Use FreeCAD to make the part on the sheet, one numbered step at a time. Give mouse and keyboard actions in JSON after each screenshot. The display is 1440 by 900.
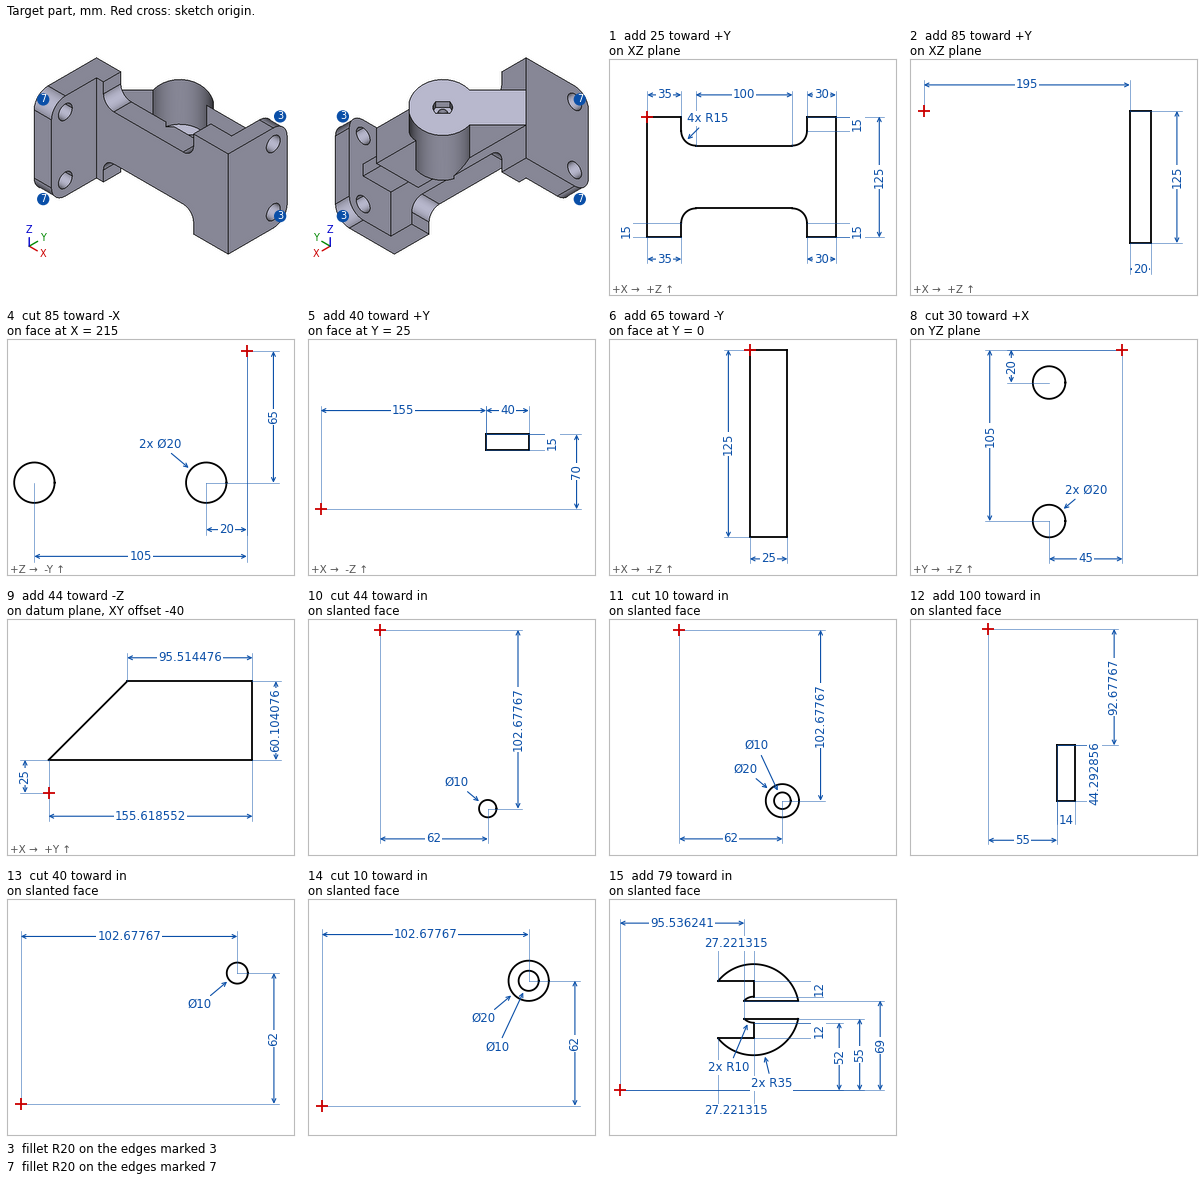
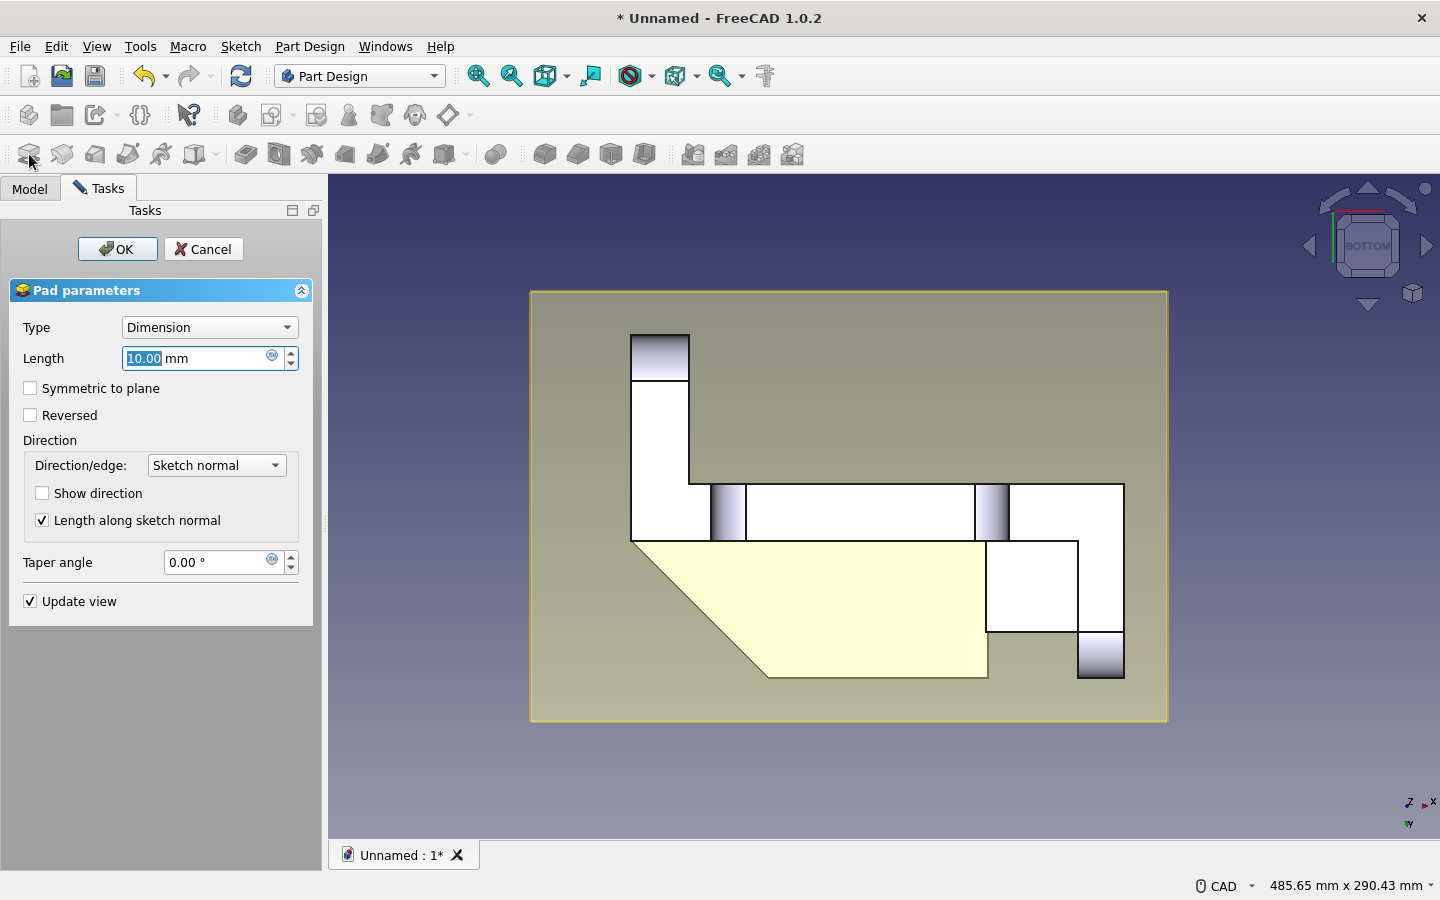
{"action": "type", "text": "44"}
{"action": "key", "text": "Tab"}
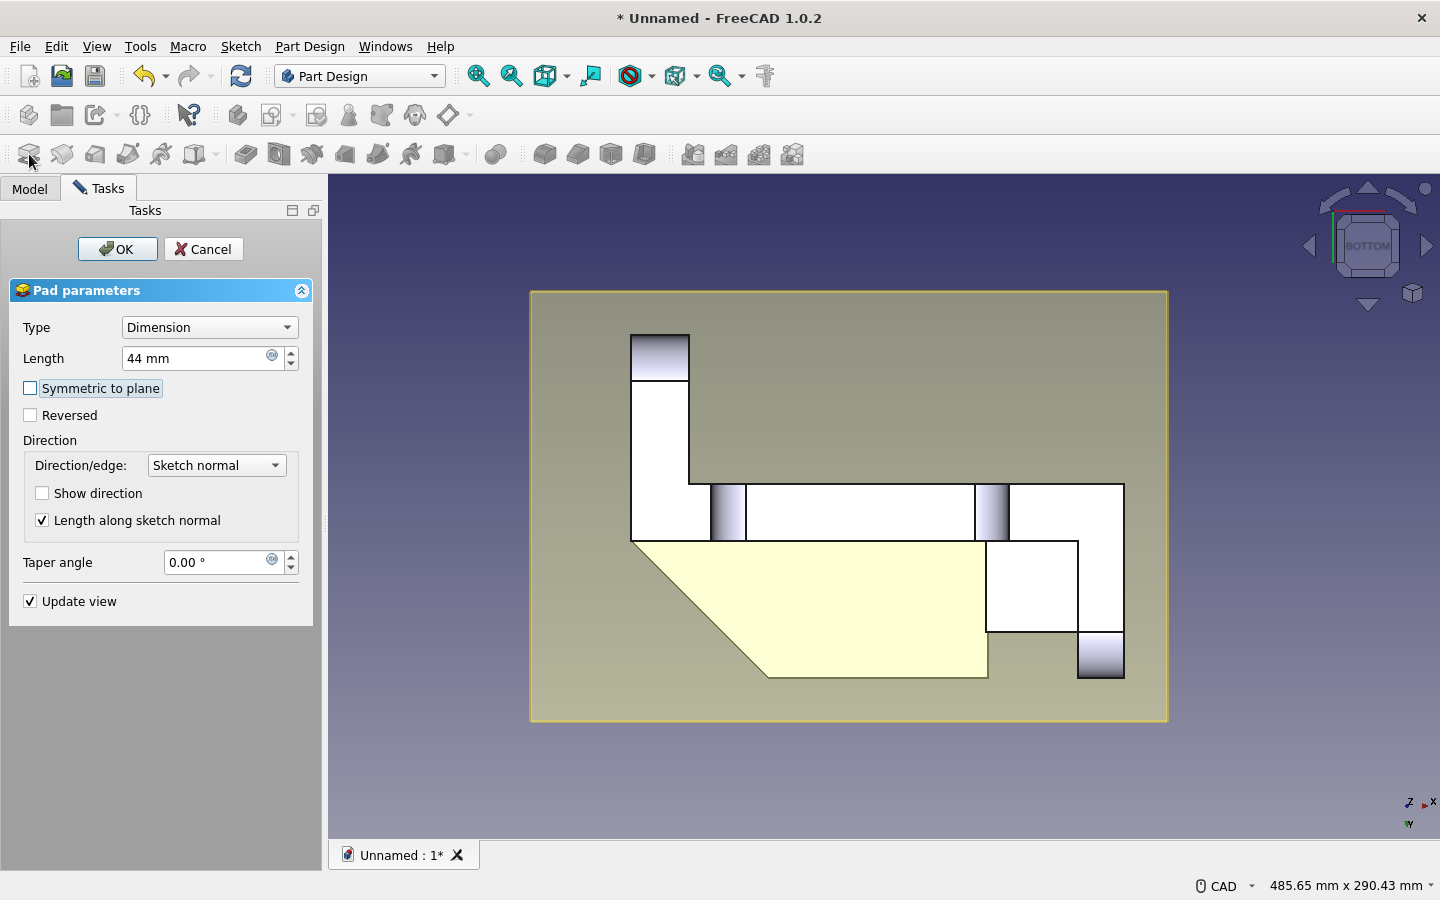
{"action": "left_click", "coordinate": [31, 415]}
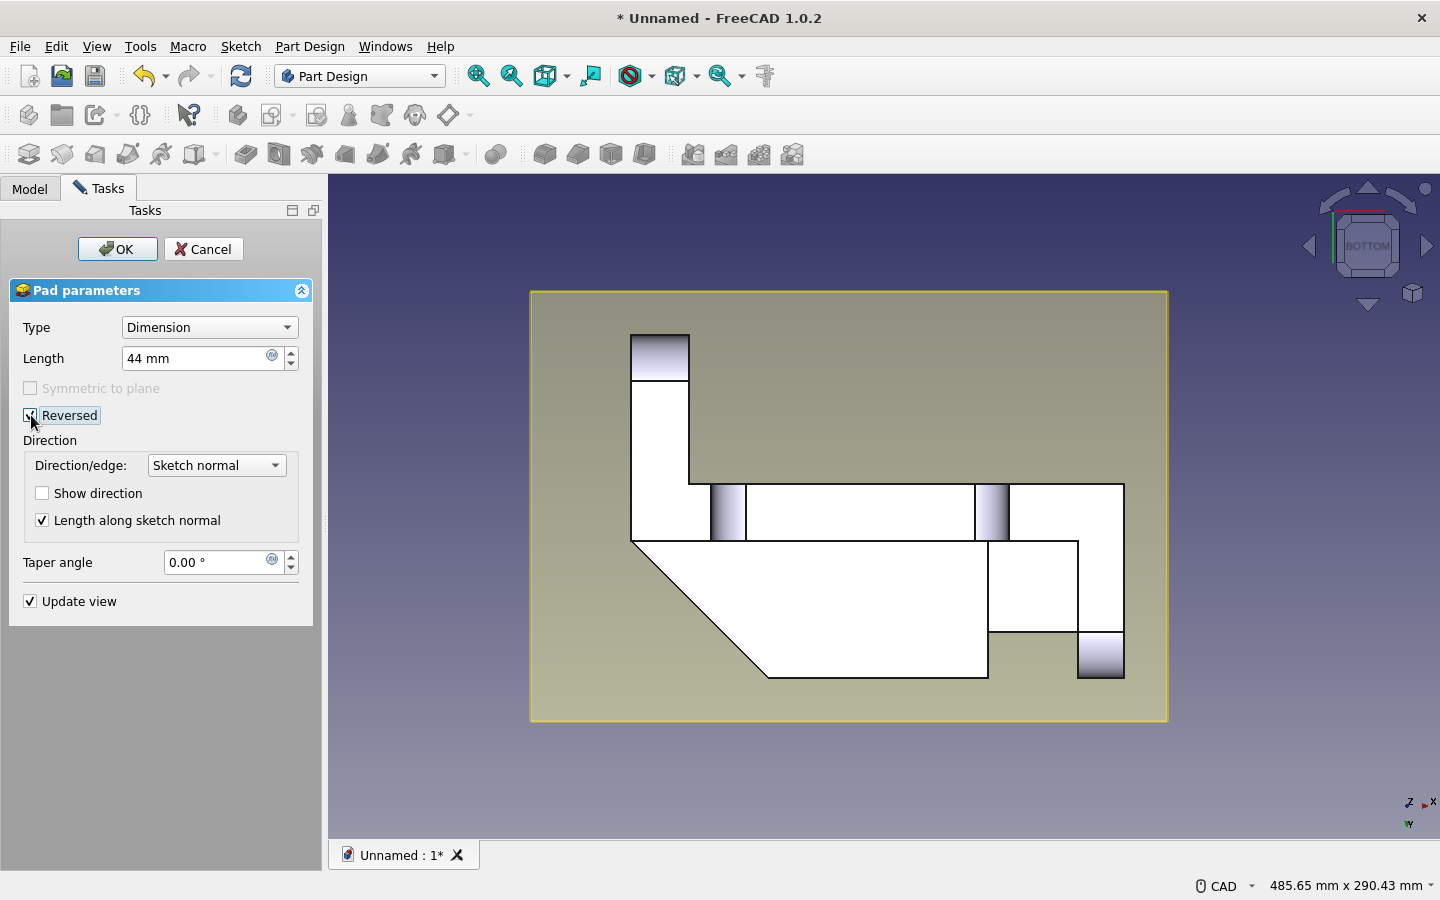
{"action": "left_click", "coordinate": [118, 249]}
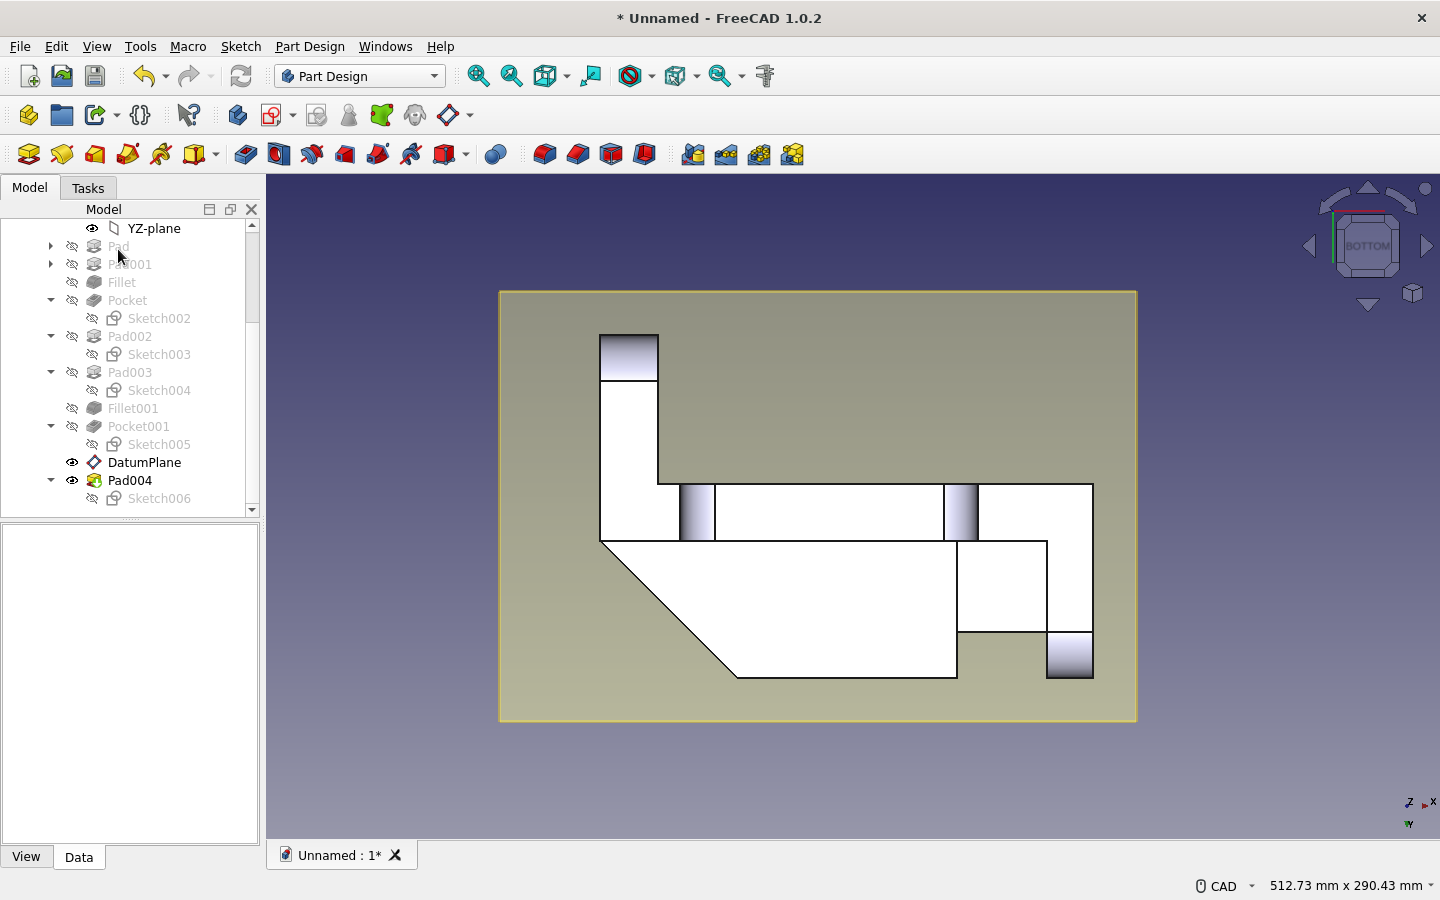
{"action": "left_click", "coordinate": [117, 462]}
{"action": "key", "text": "space"}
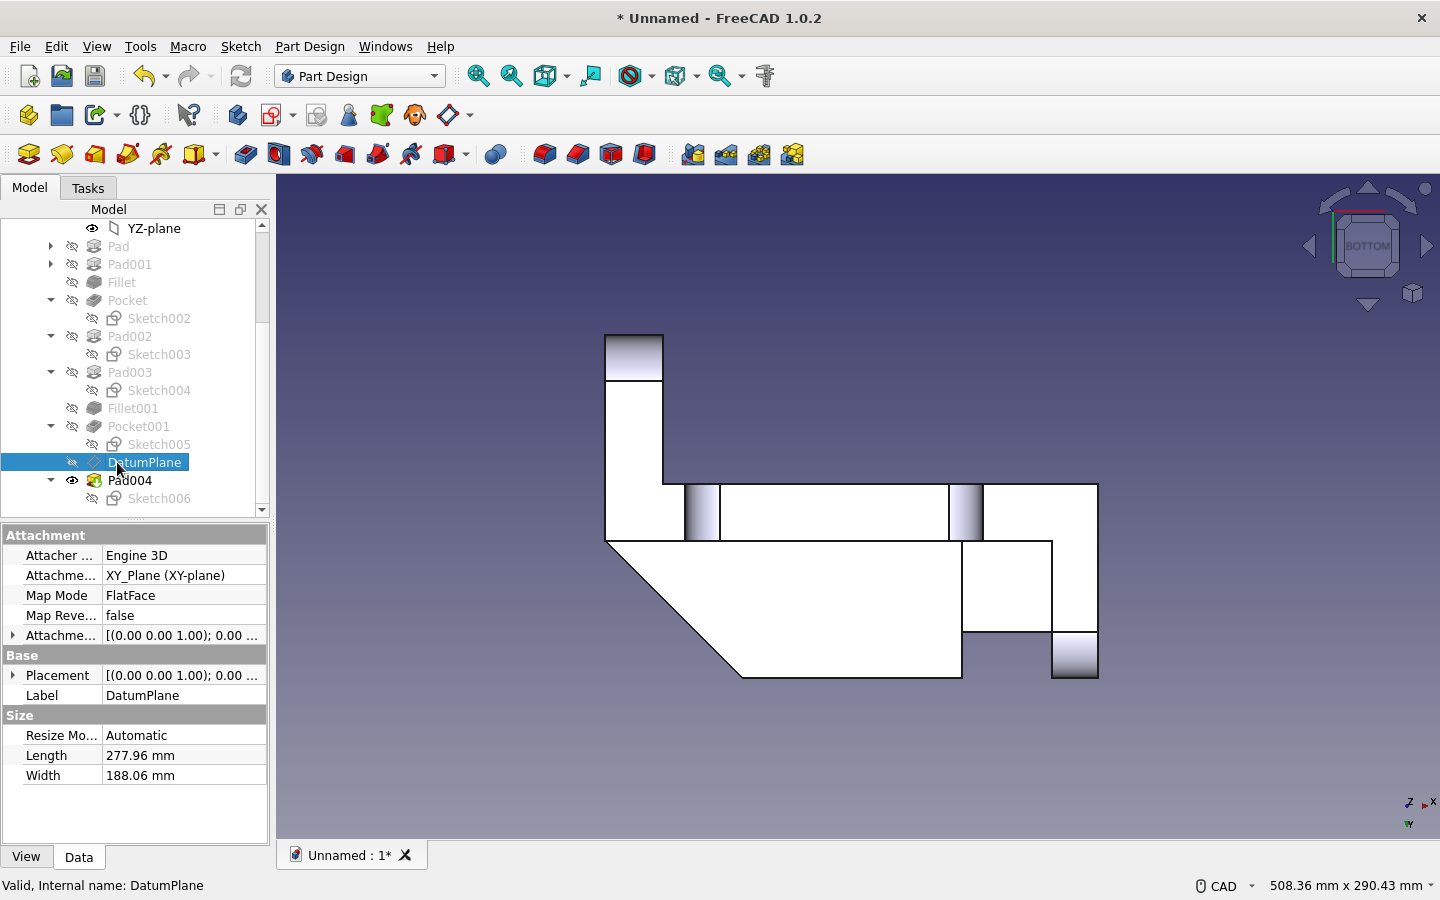
{"action": "key", "text": "6"}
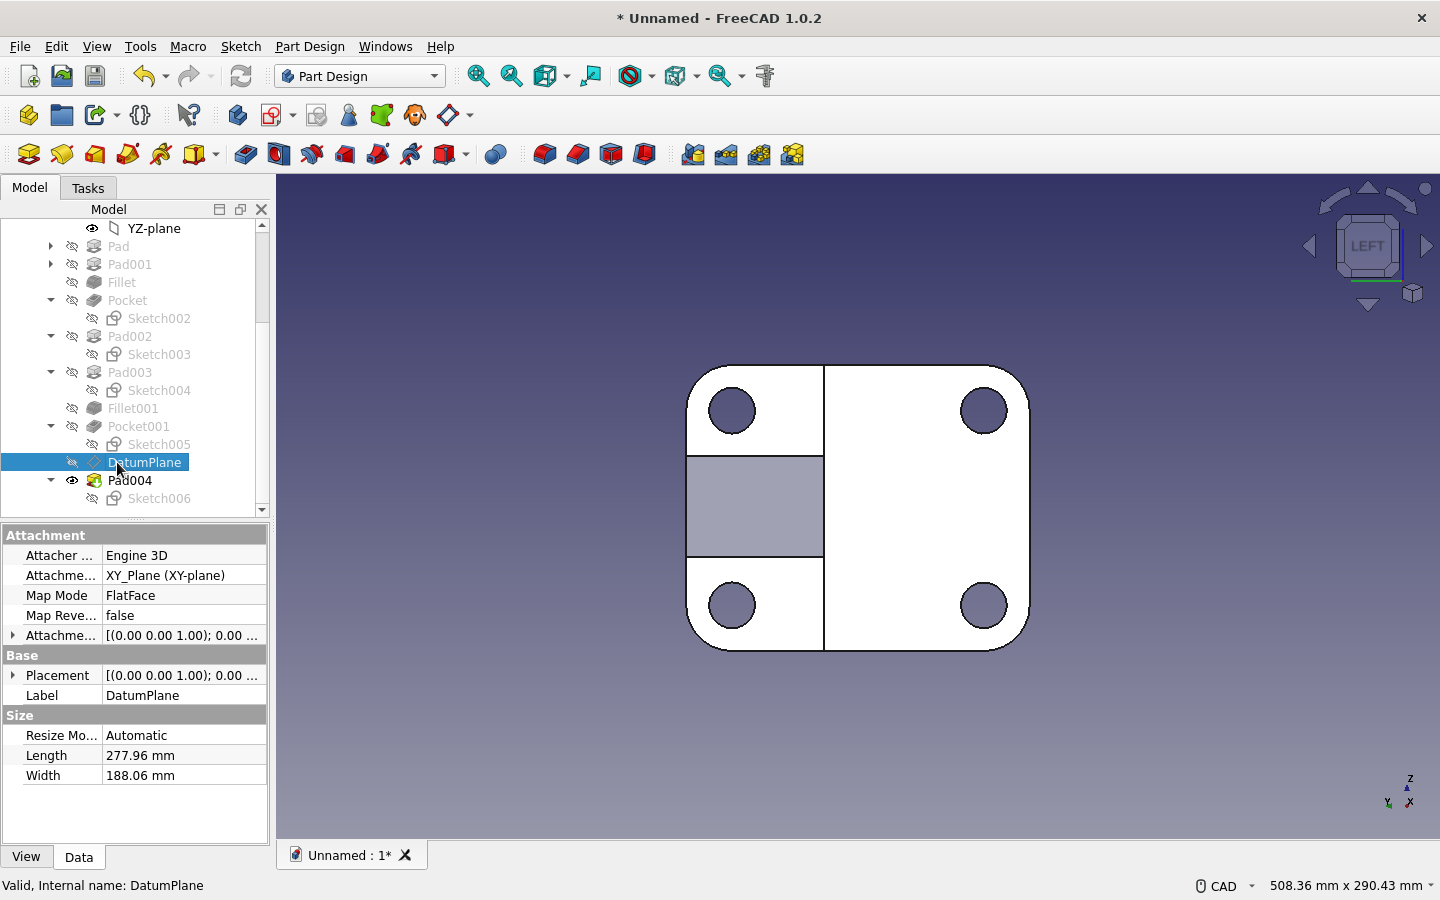
{"action": "left_click", "coordinate": [479, 76]}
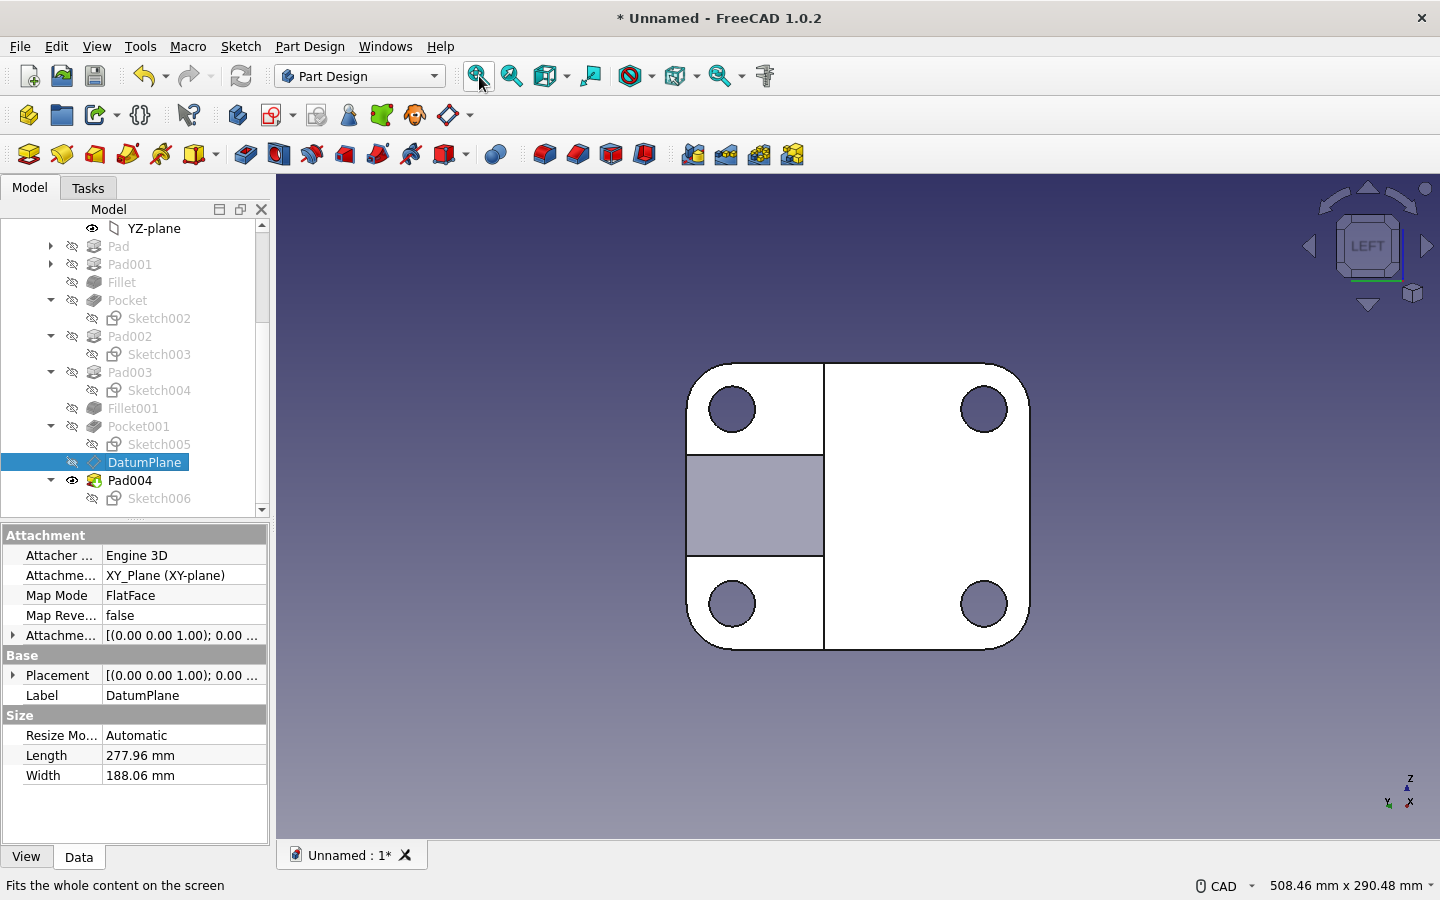
{"action": "left_click", "coordinate": [735, 504]}